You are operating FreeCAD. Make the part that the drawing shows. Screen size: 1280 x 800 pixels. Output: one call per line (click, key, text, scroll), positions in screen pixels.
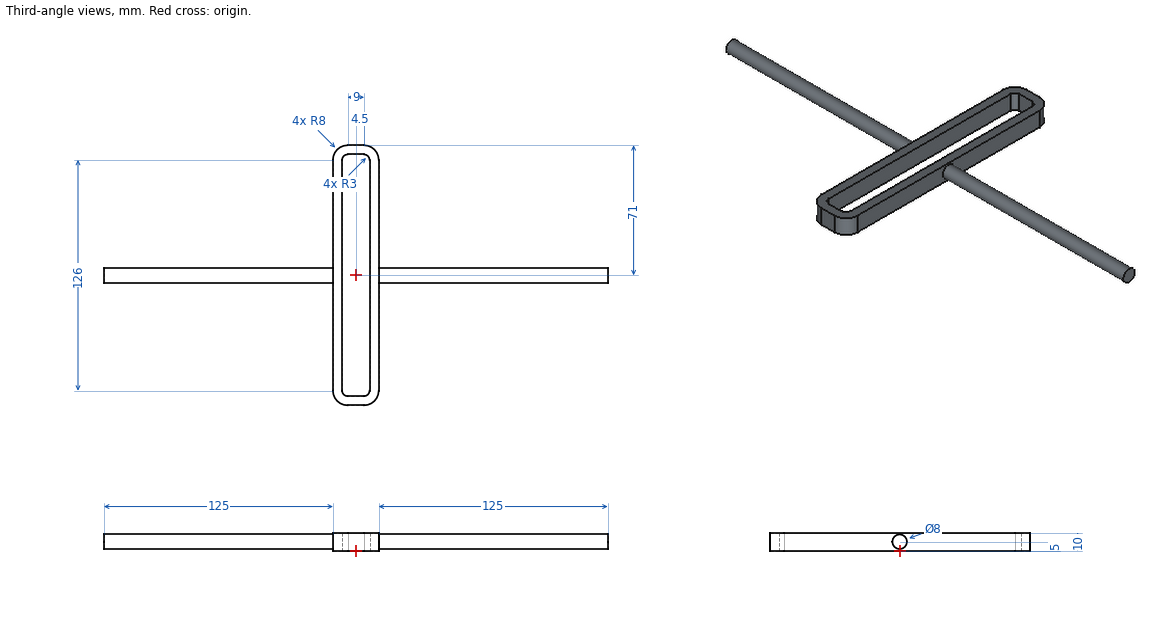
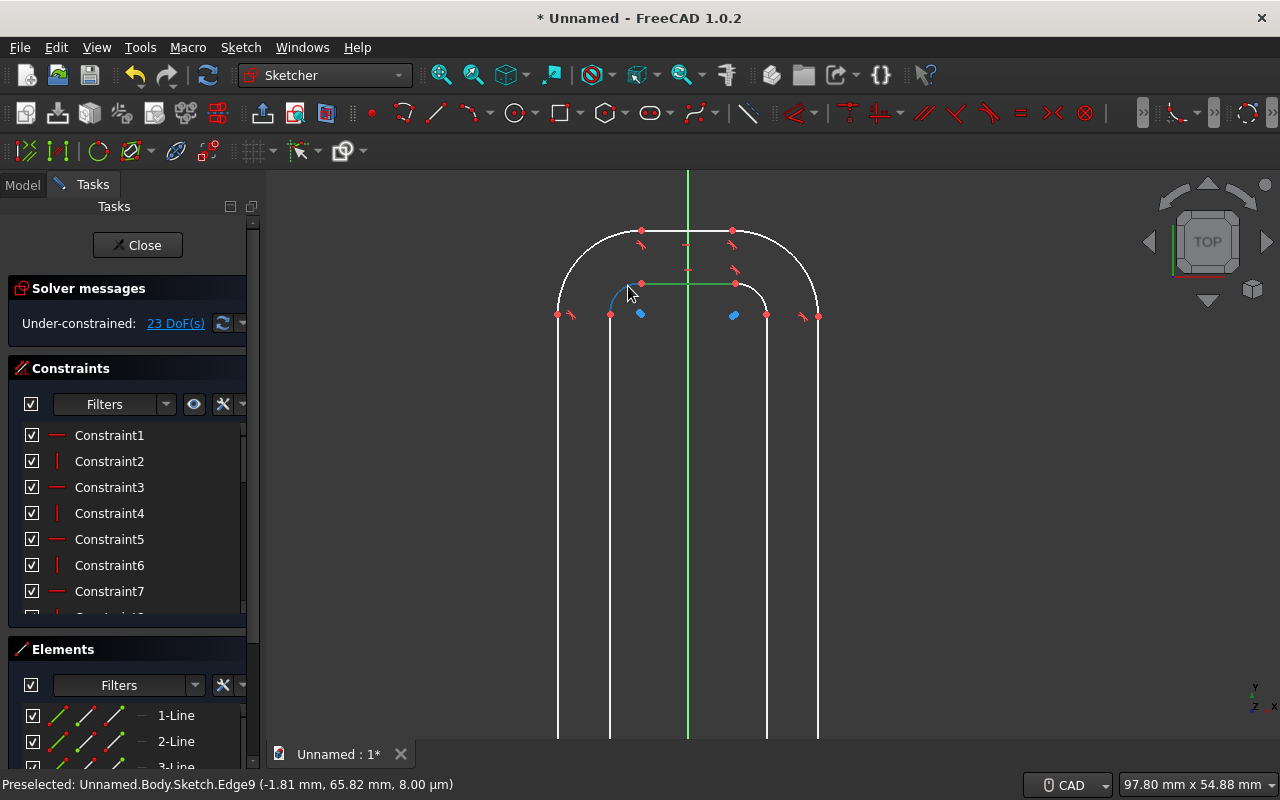
click(627, 286)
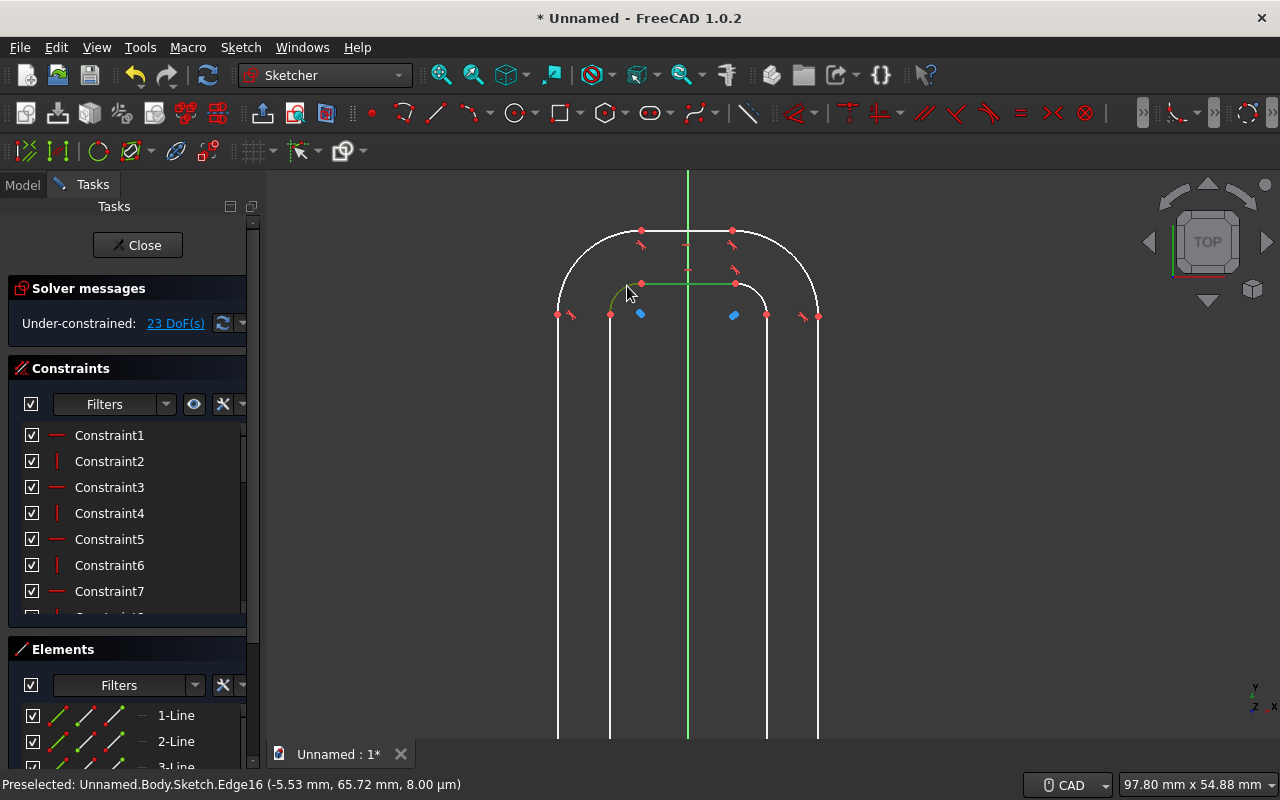
click(990, 114)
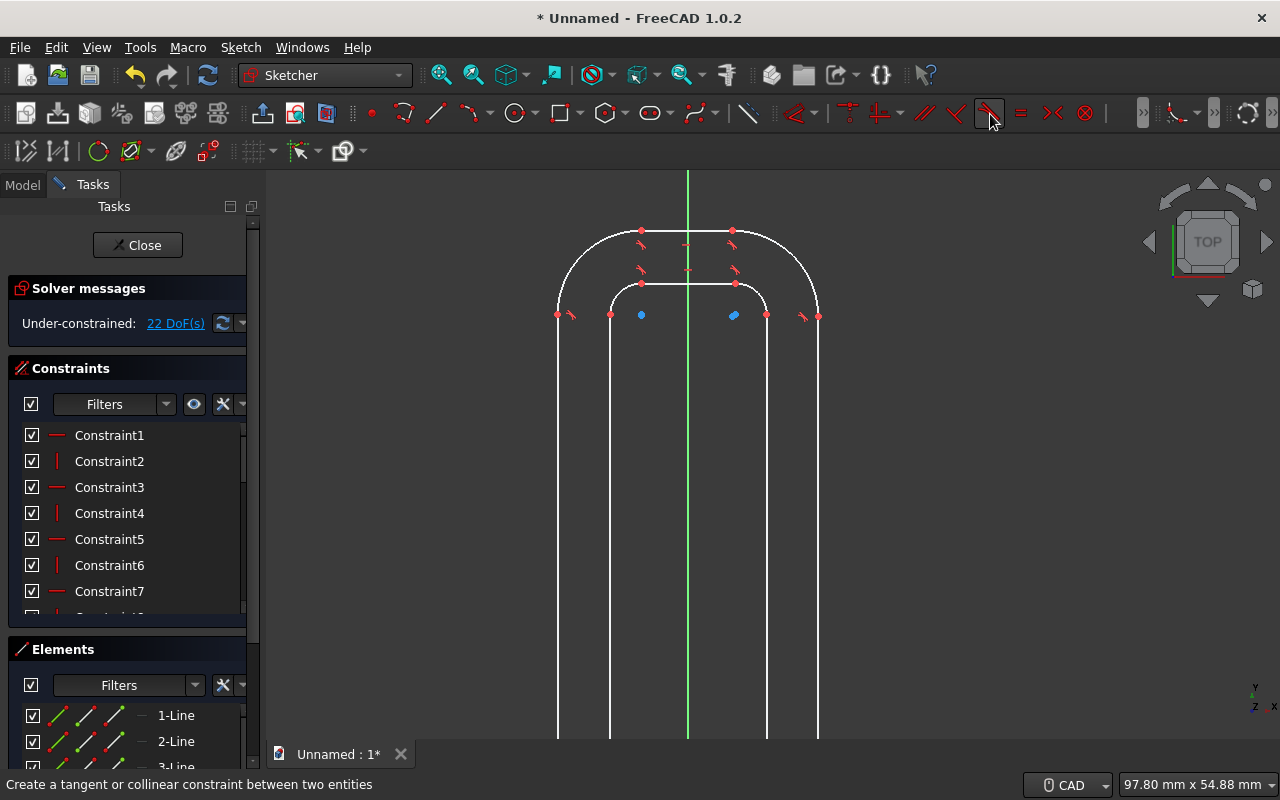
scroll(710, 287, down, 7)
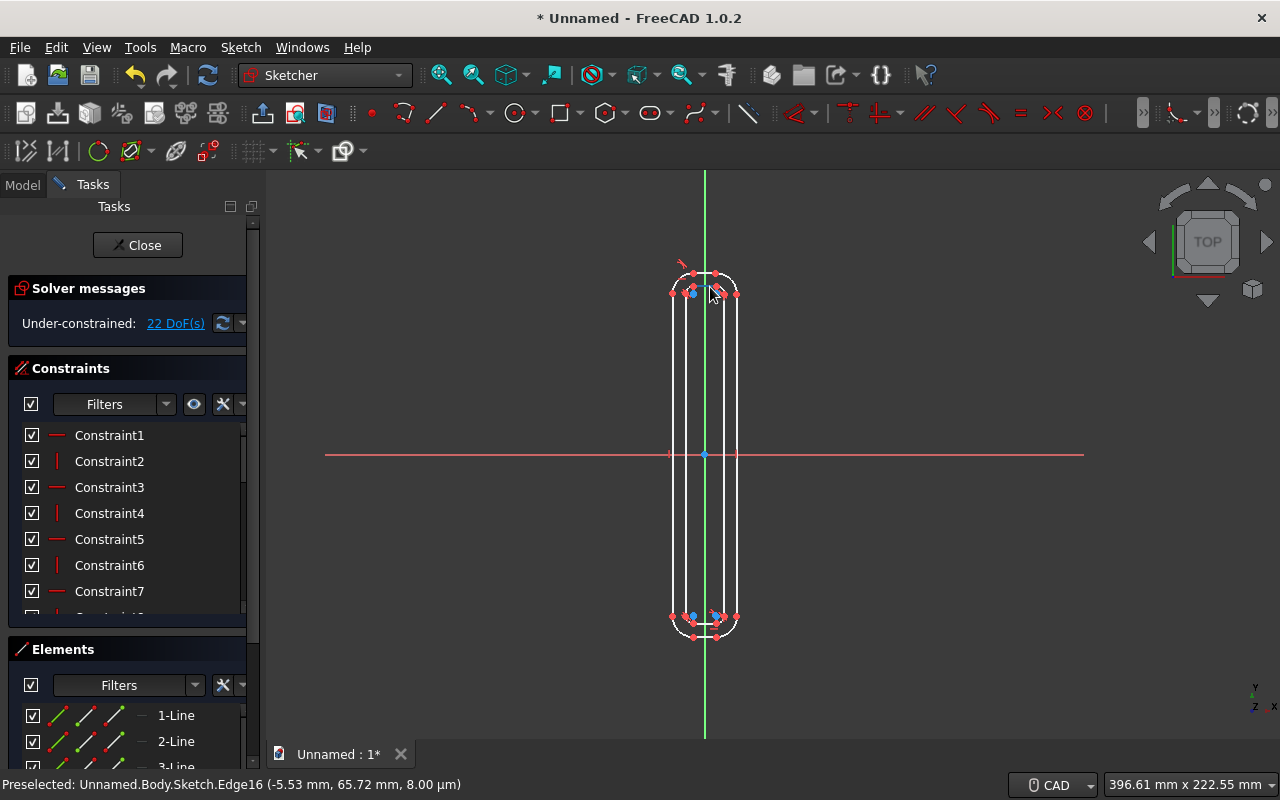
click(724, 391)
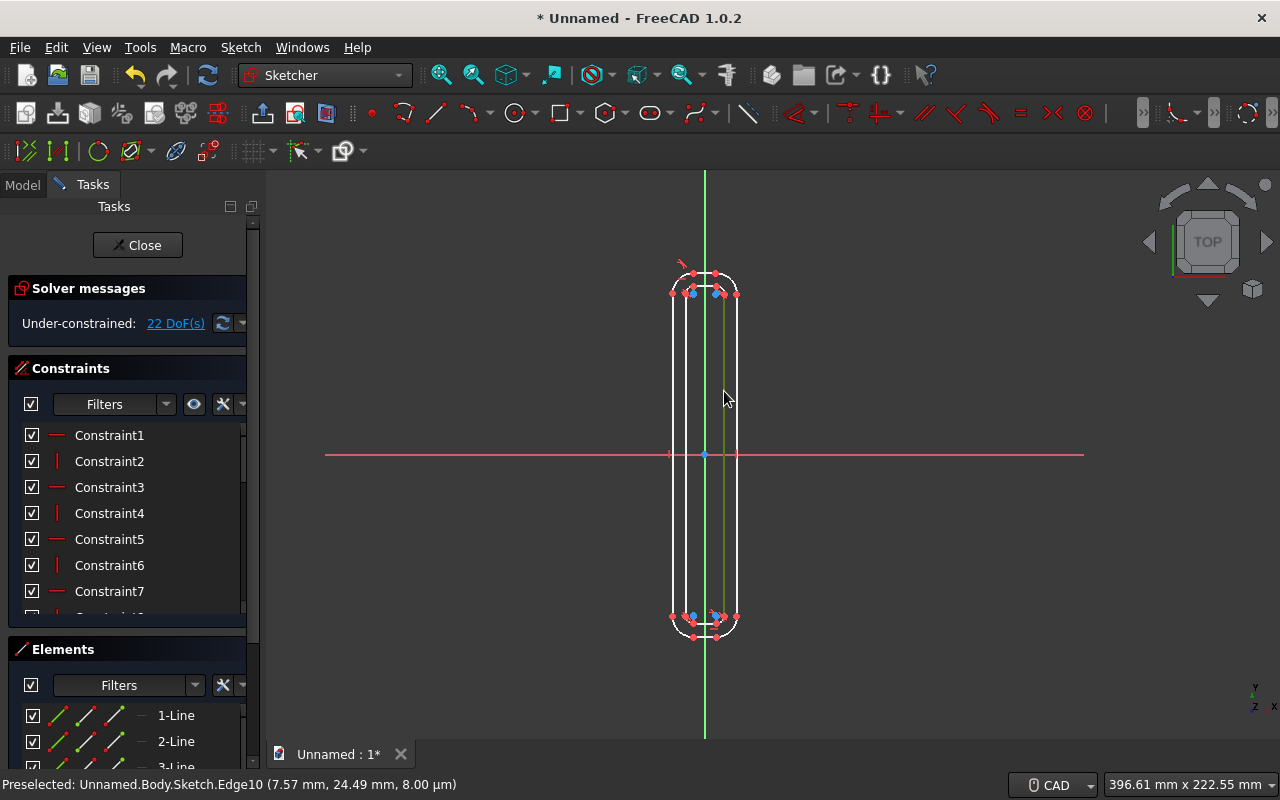
scroll(722, 289, up, 5)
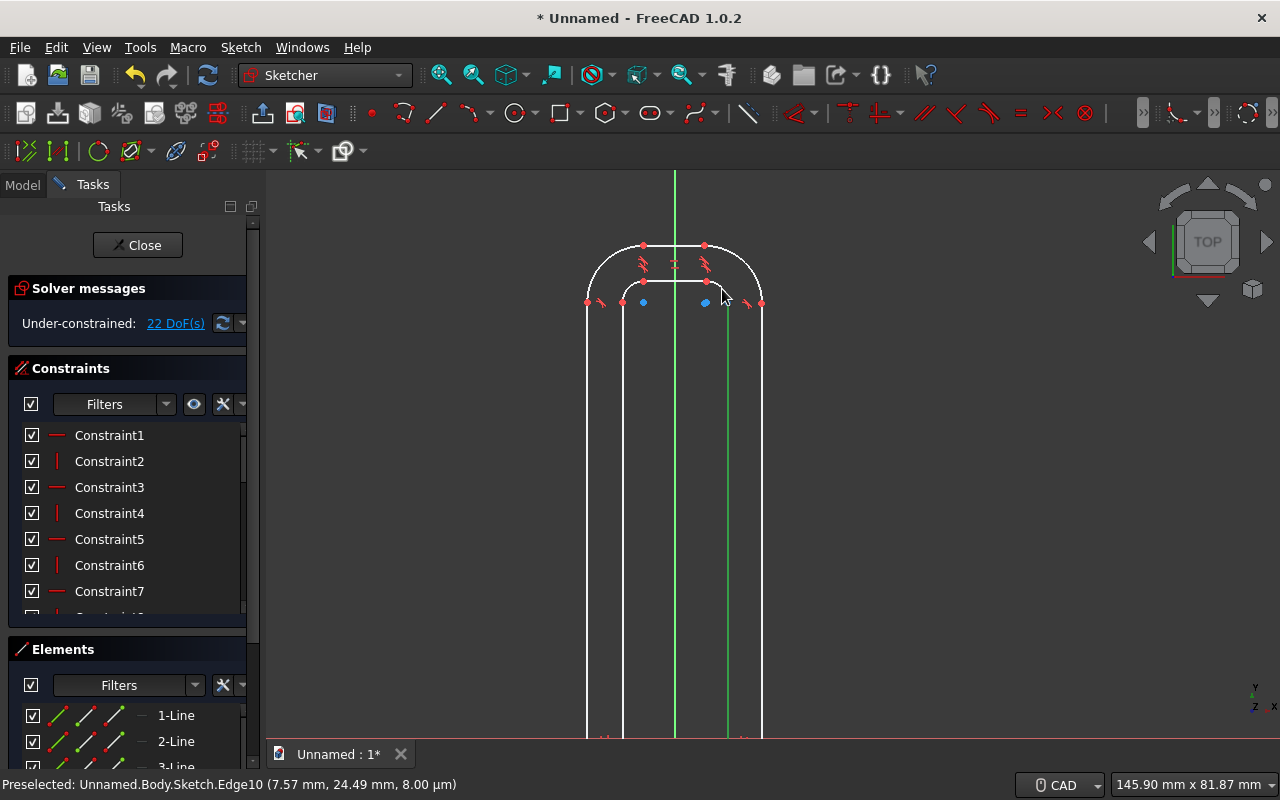
click(722, 287)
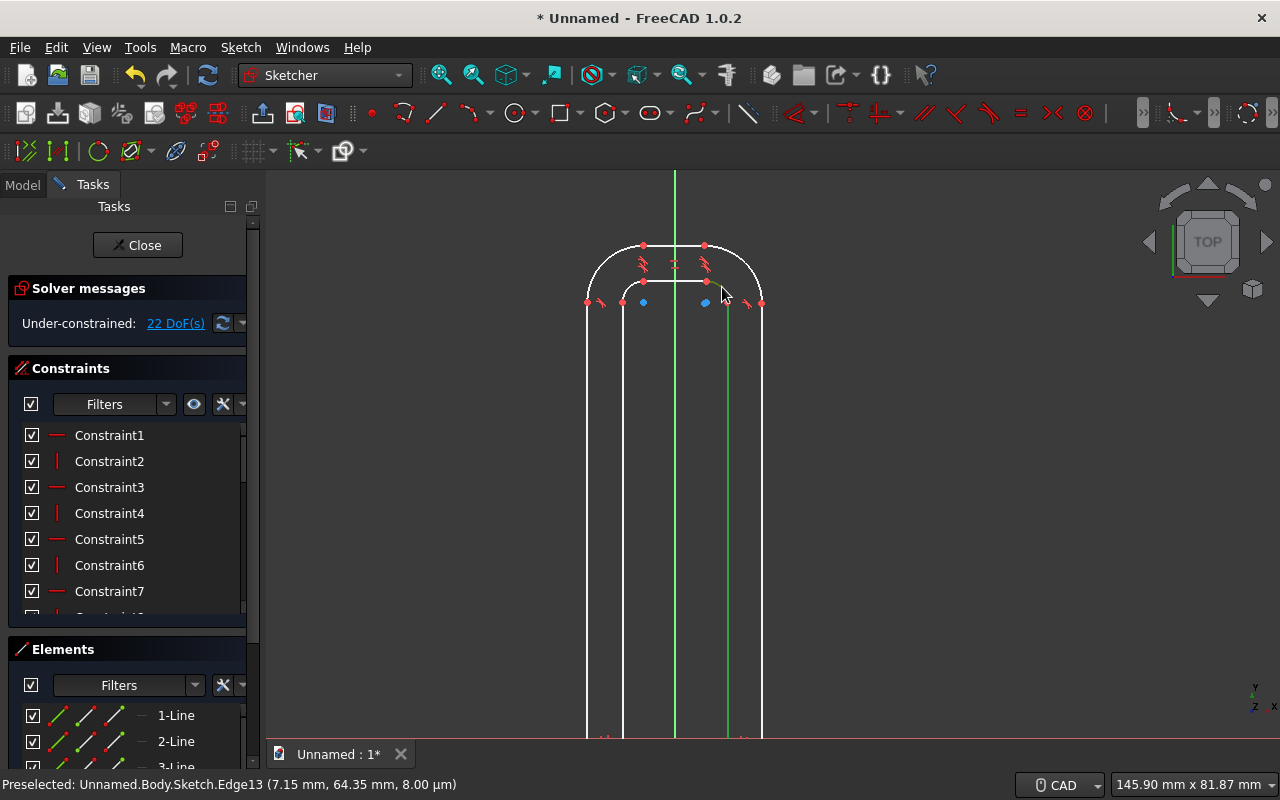
click(990, 114)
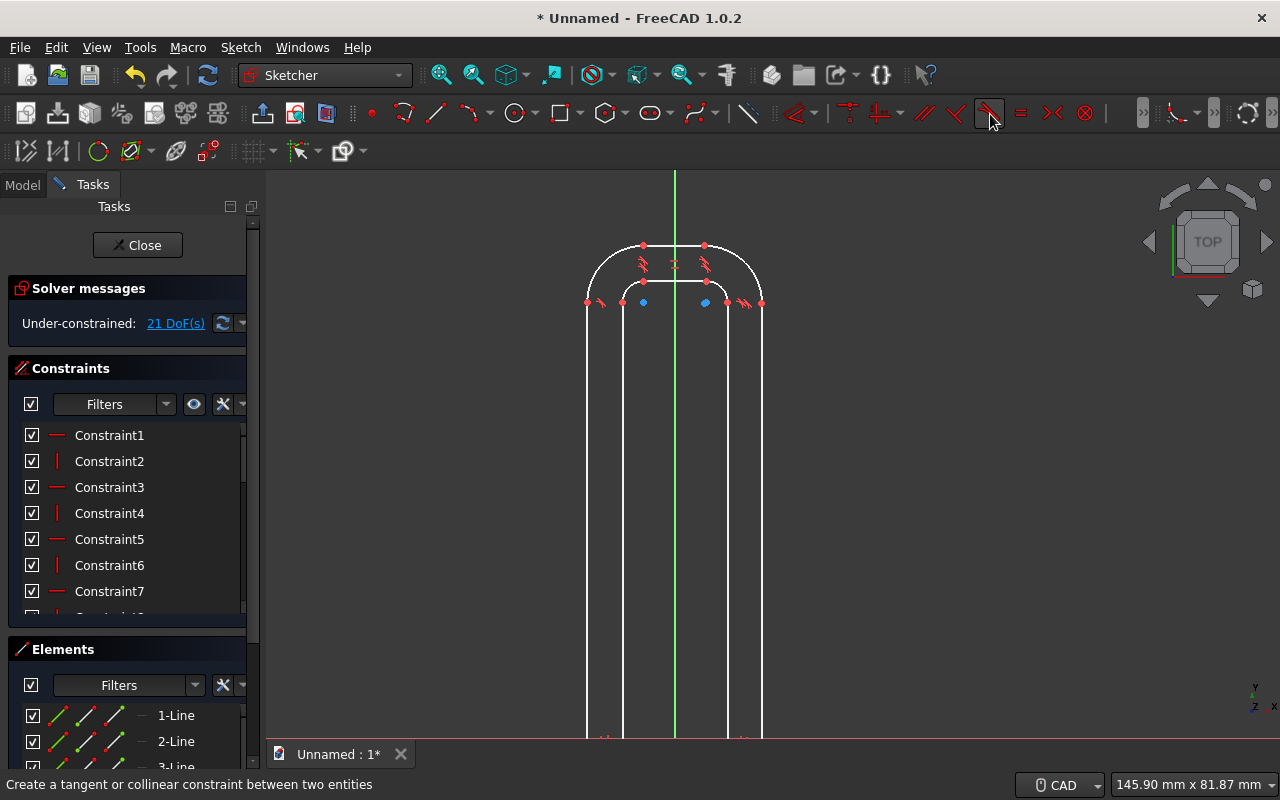
click(728, 565)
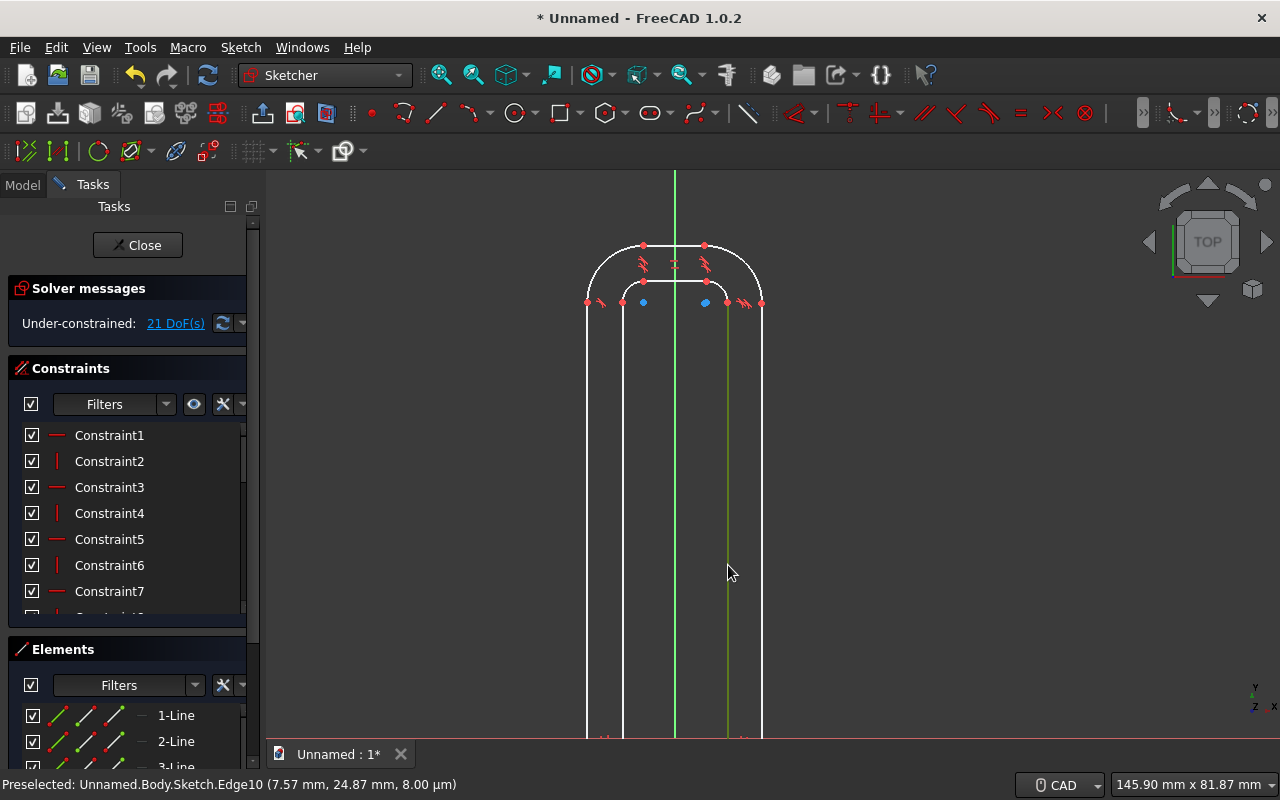
scroll(722, 289, down, 5)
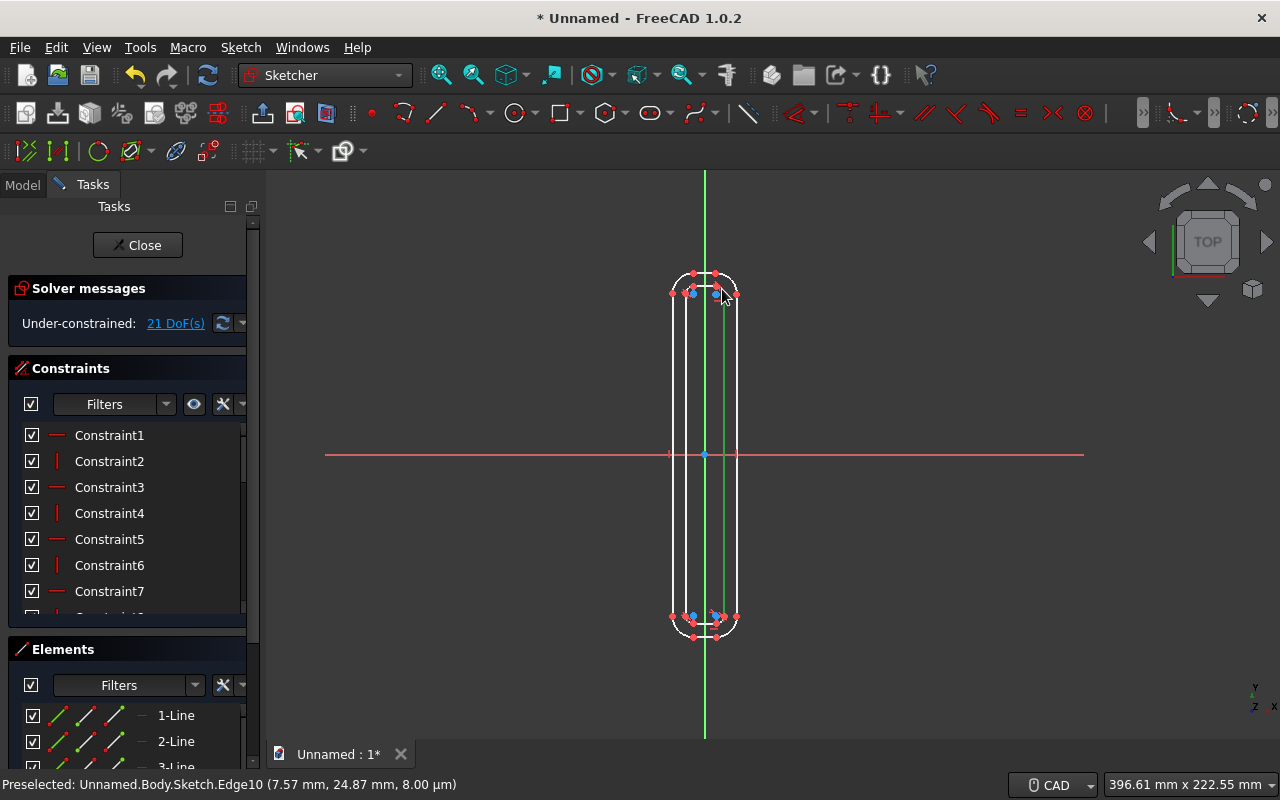
scroll(720, 623, up, 7)